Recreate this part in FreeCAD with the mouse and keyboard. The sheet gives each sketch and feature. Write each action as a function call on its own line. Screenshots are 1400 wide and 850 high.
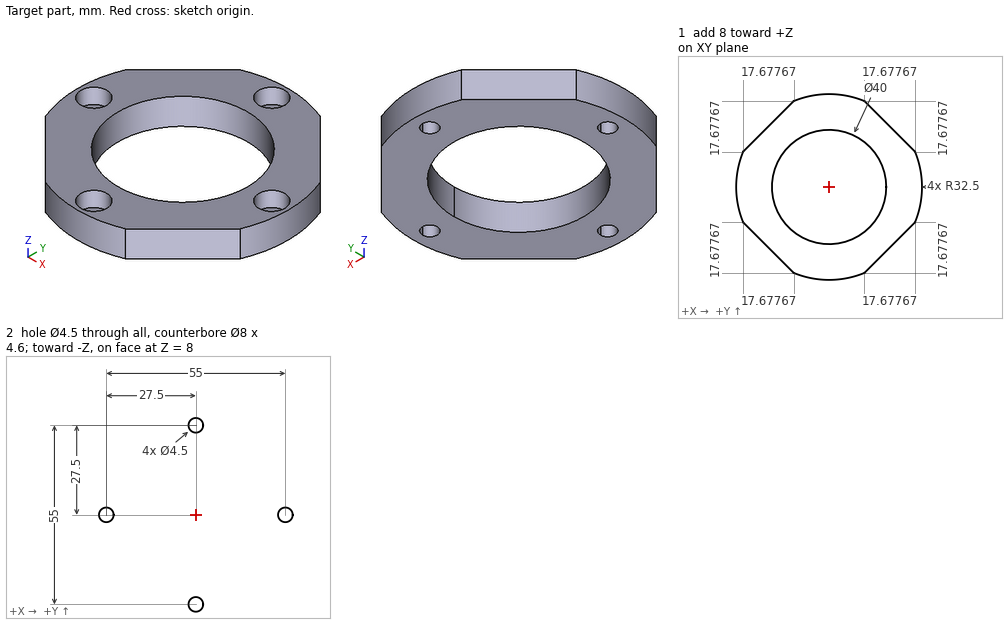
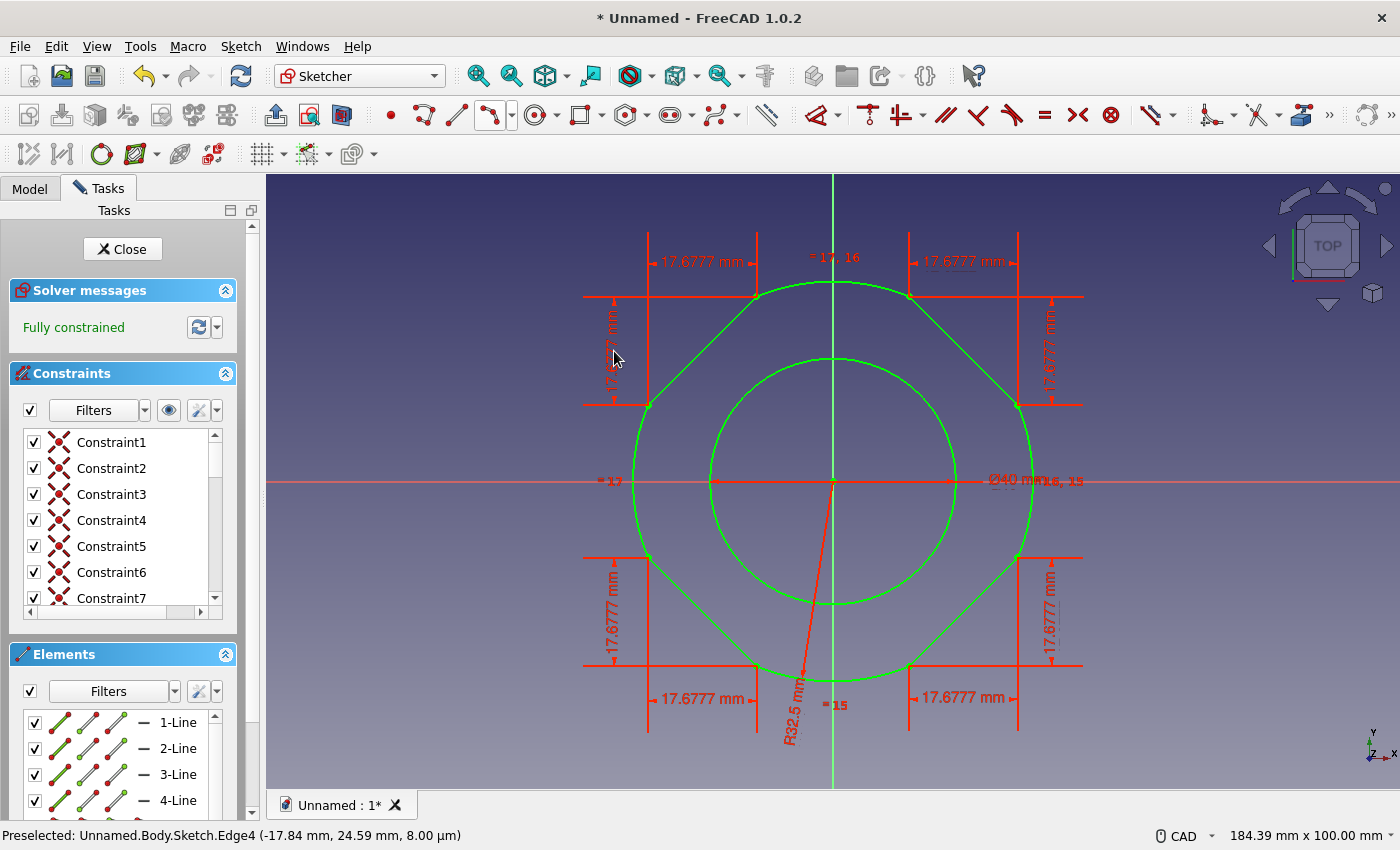
click(123, 249)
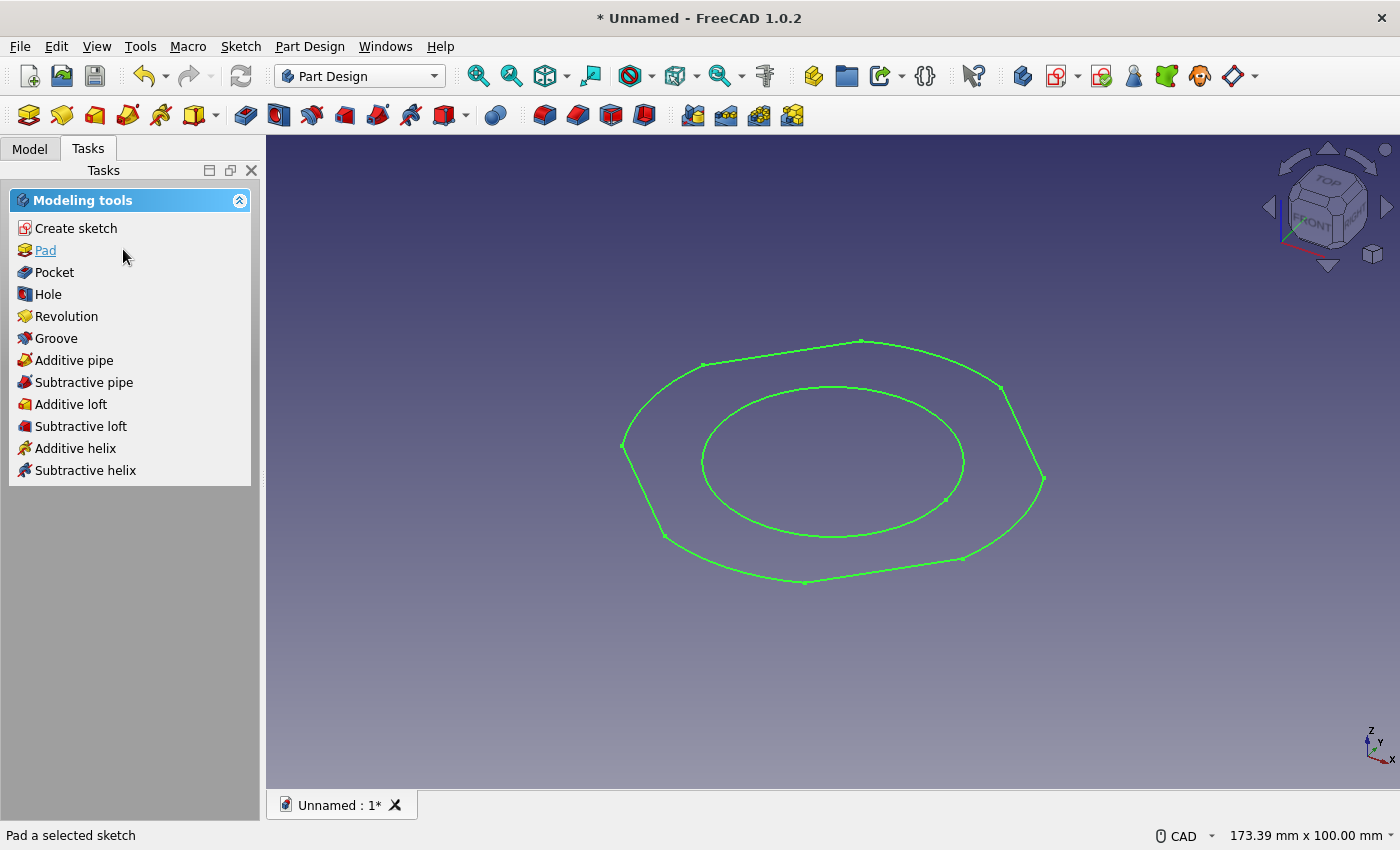
click(29, 116)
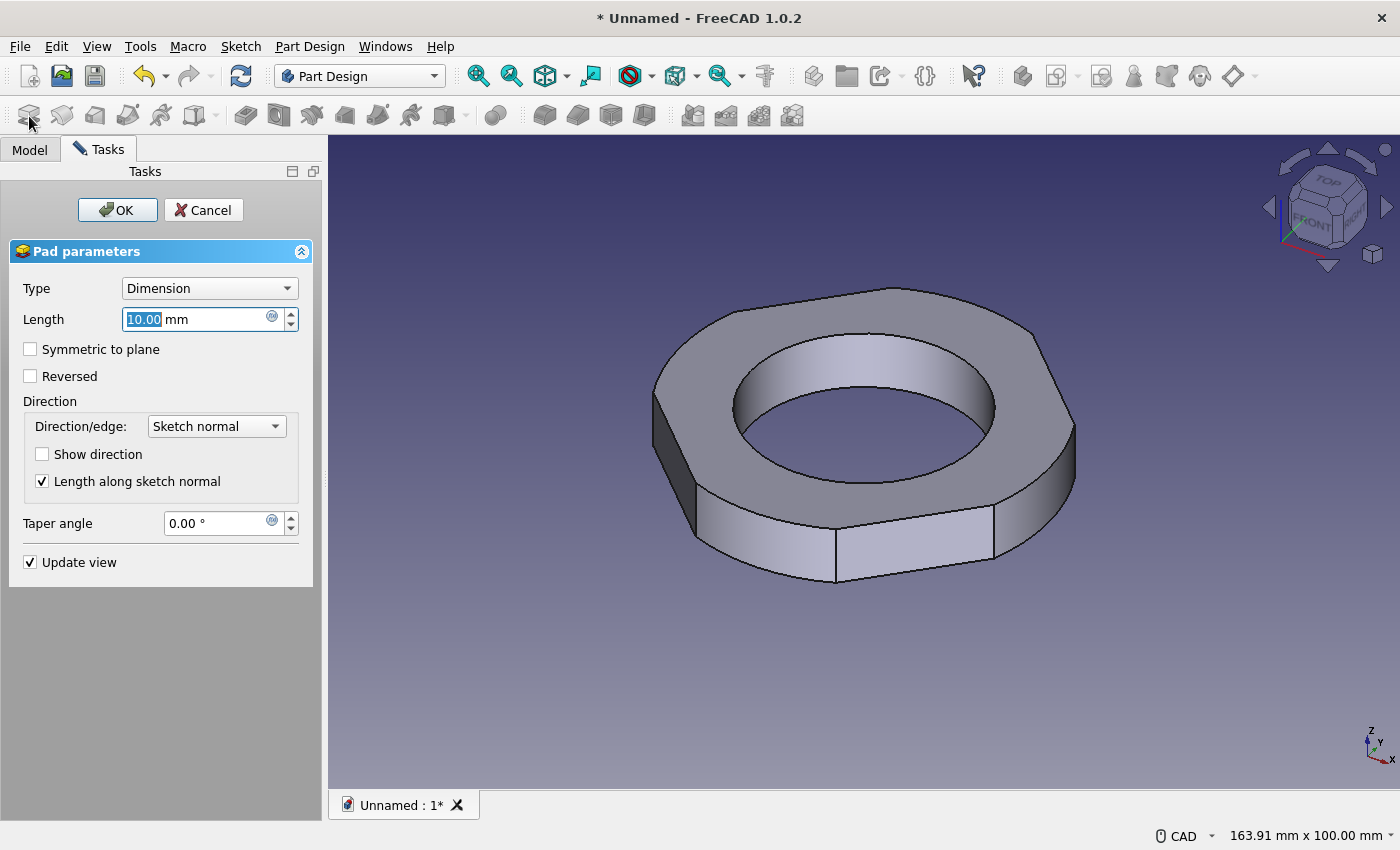
text(8)
key(Tab)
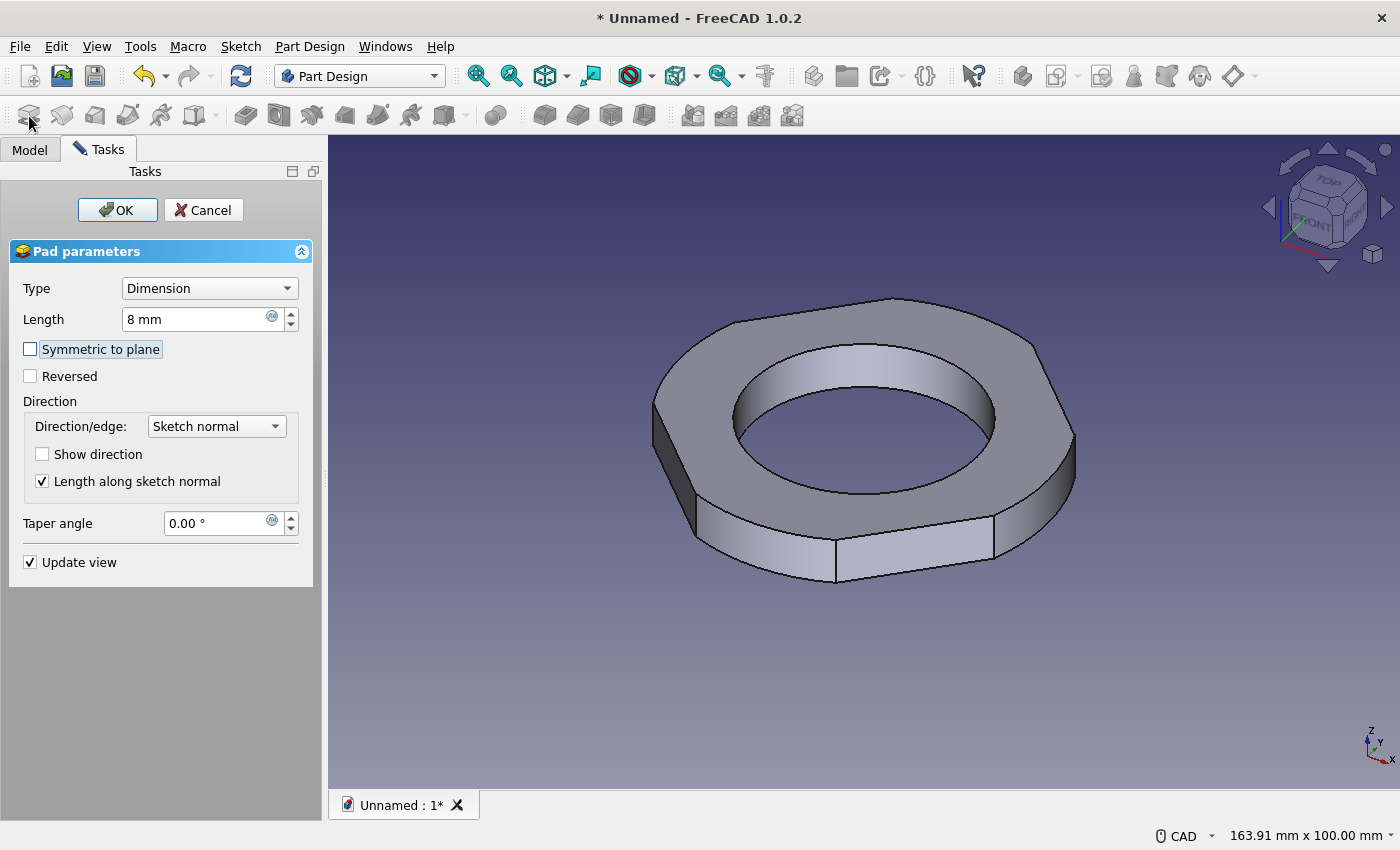
click(118, 210)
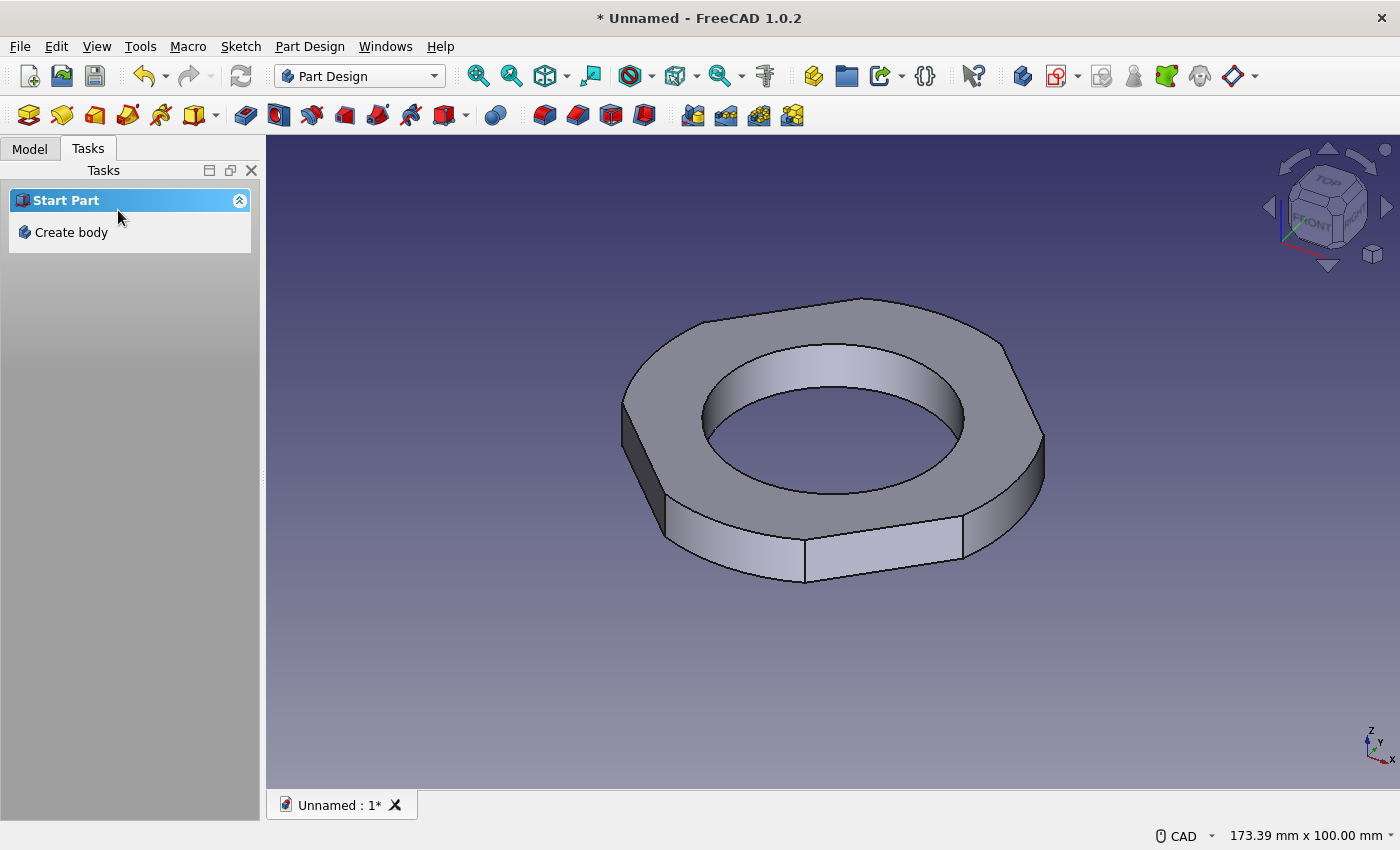
click(991, 470)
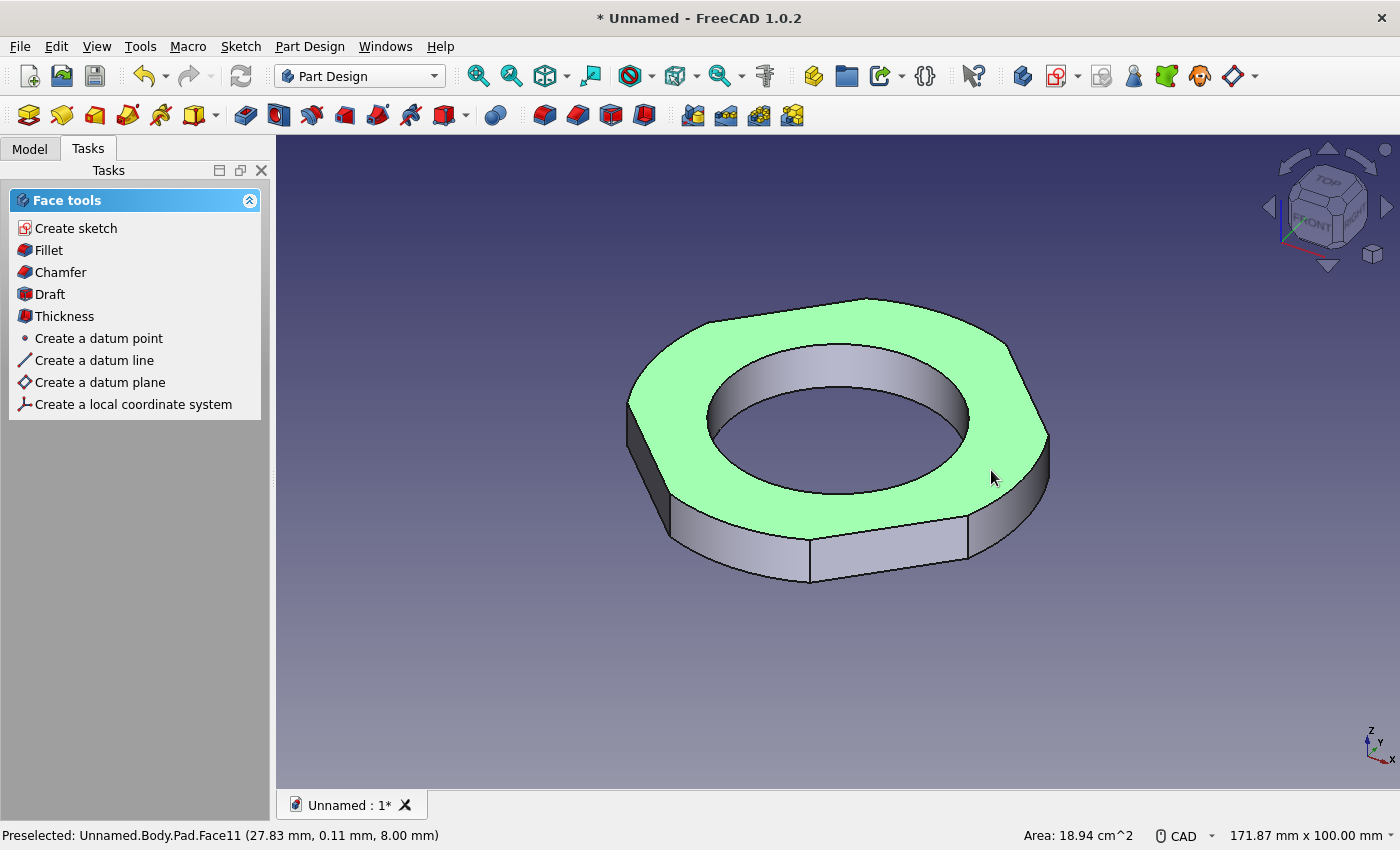
click(1056, 76)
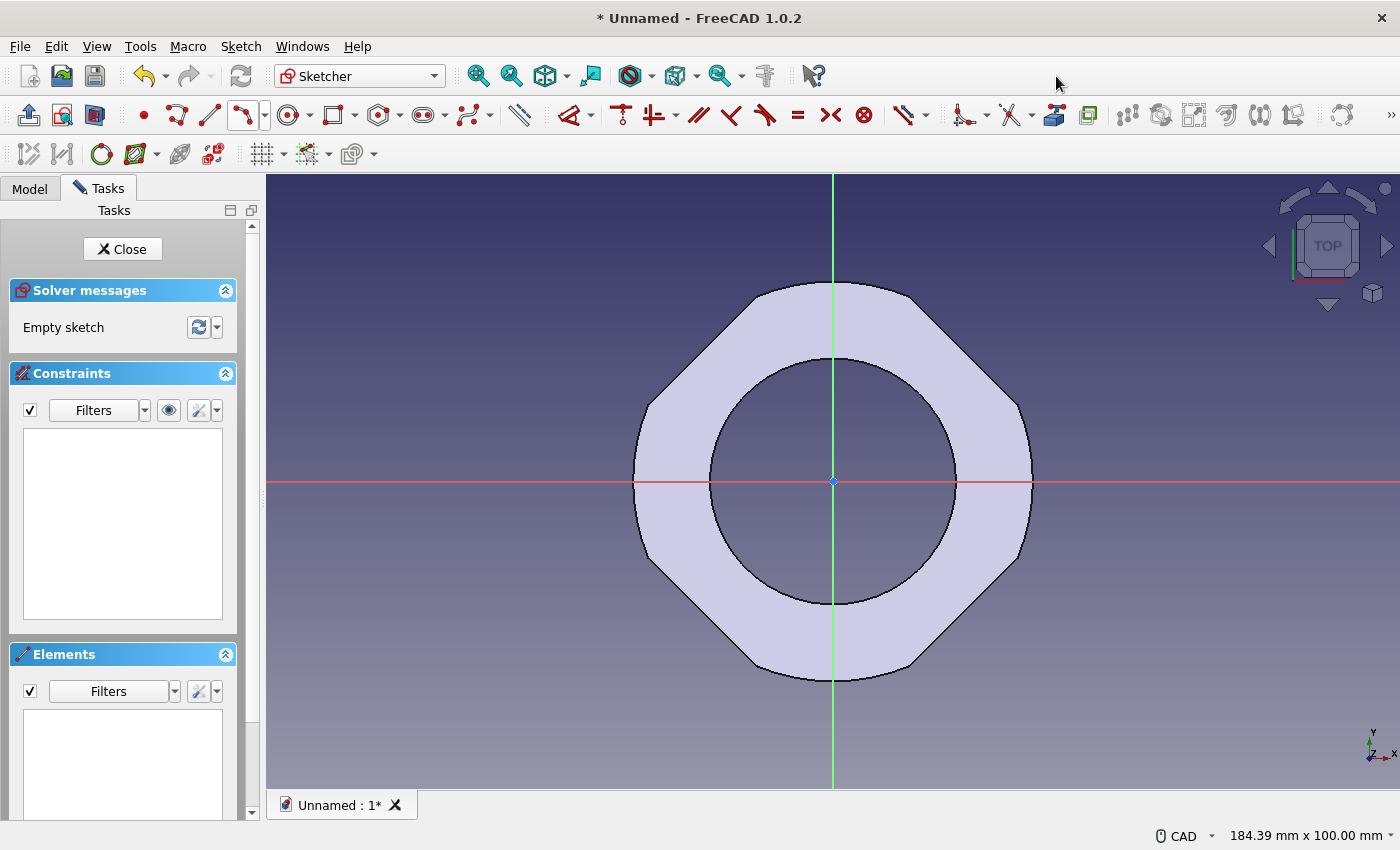
click(288, 116)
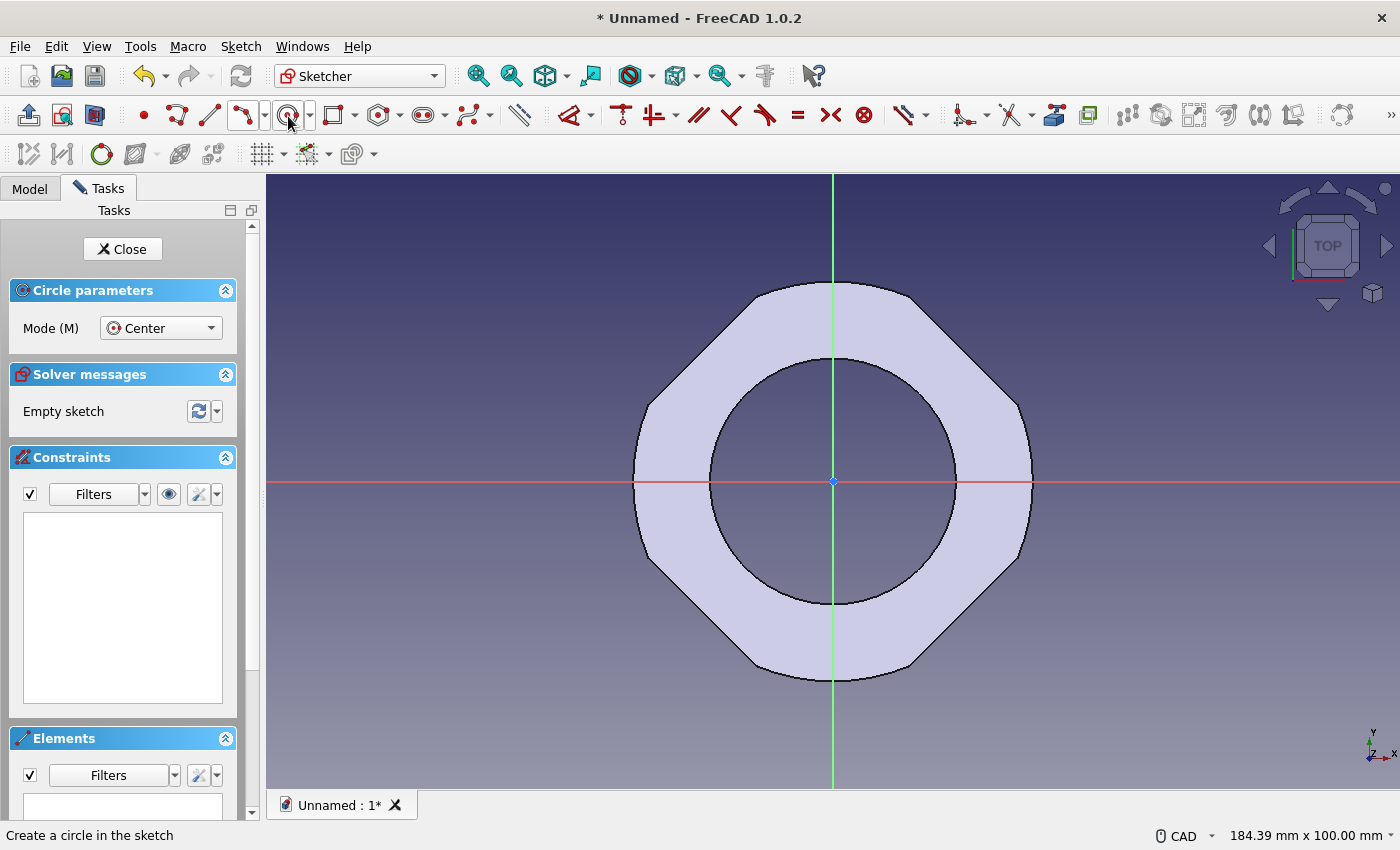
scroll(833, 312, up, 3)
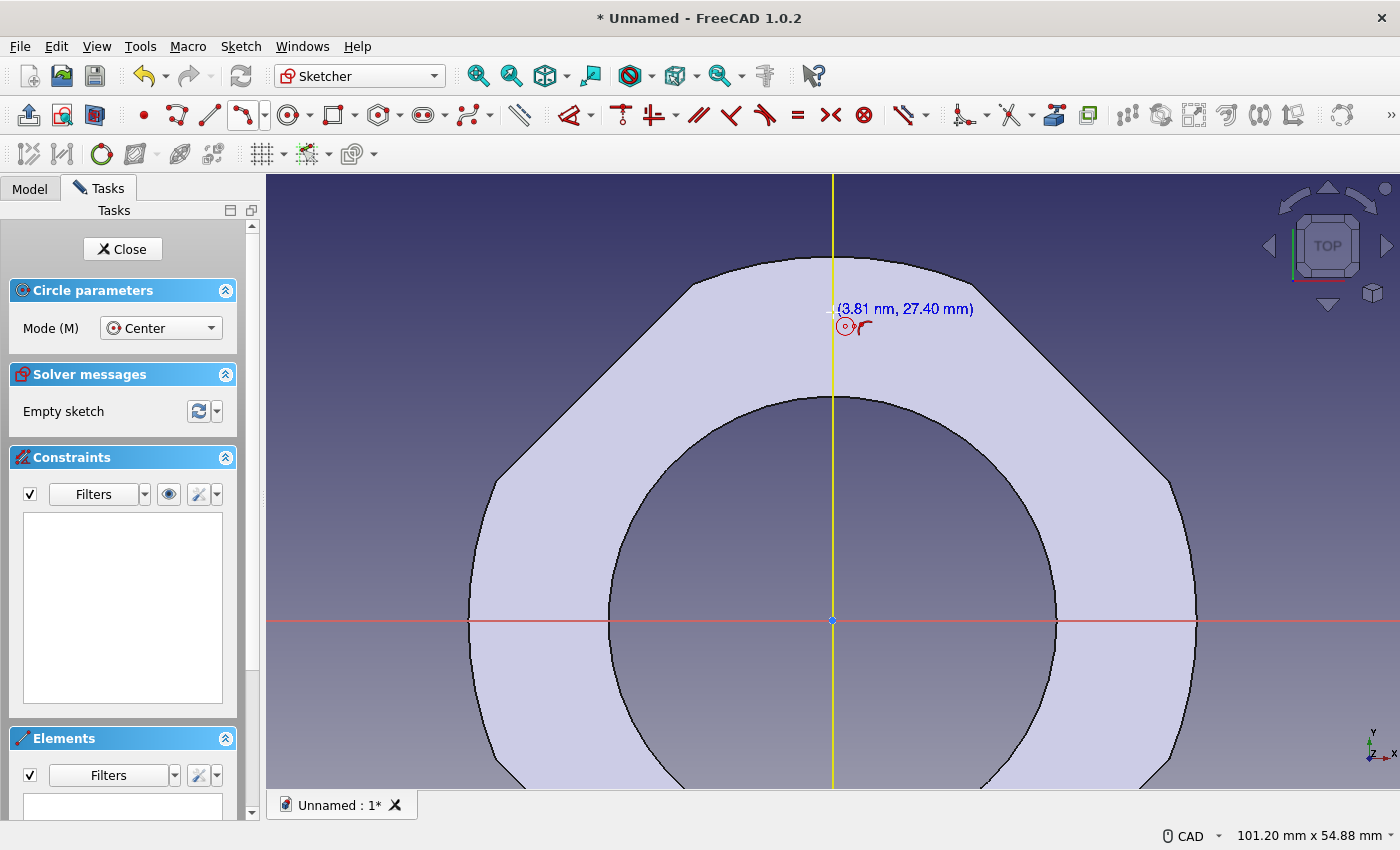
click(833, 312)
move(850, 295)